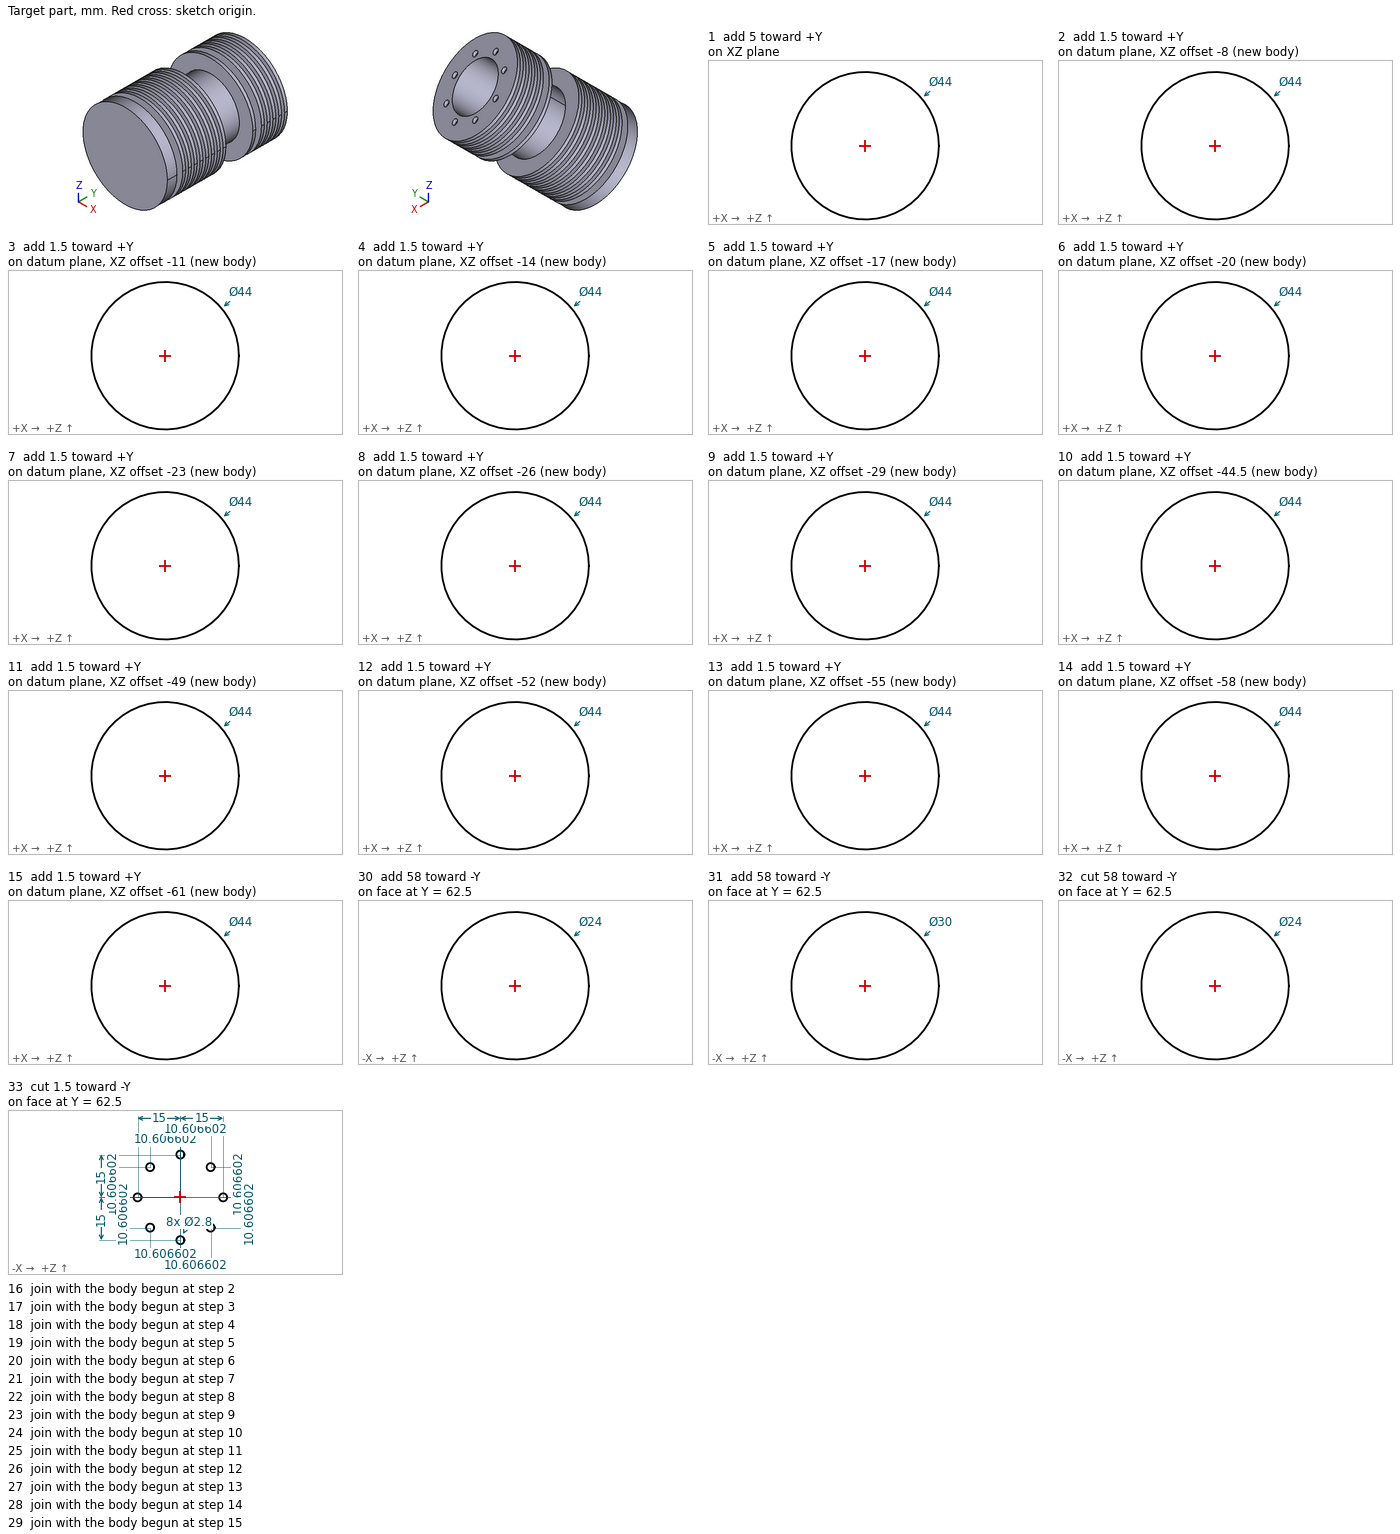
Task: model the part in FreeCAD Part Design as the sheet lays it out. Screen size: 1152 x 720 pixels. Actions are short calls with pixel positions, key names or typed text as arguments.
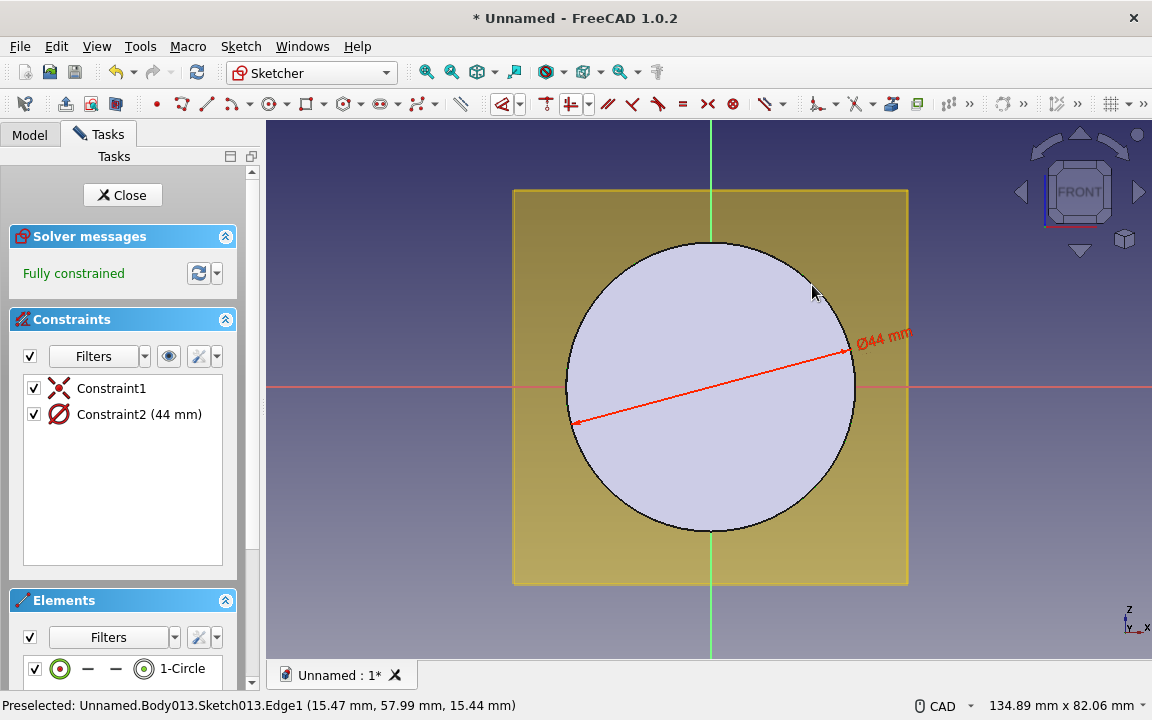
click(123, 195)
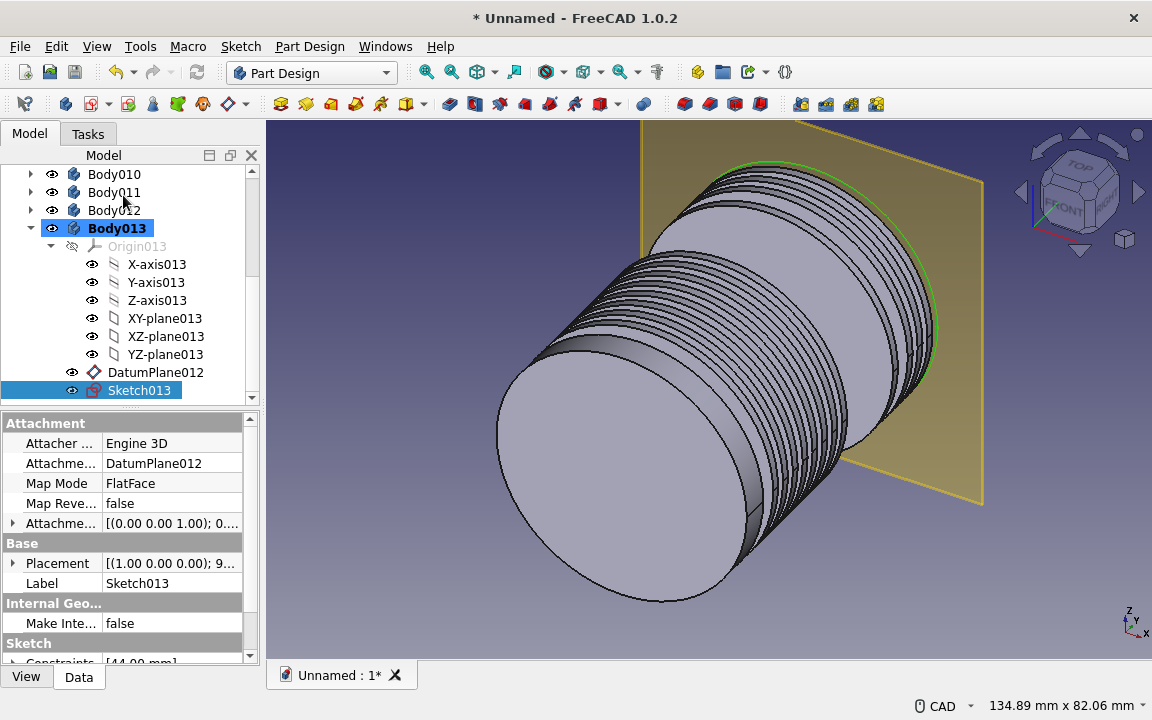
click(281, 104)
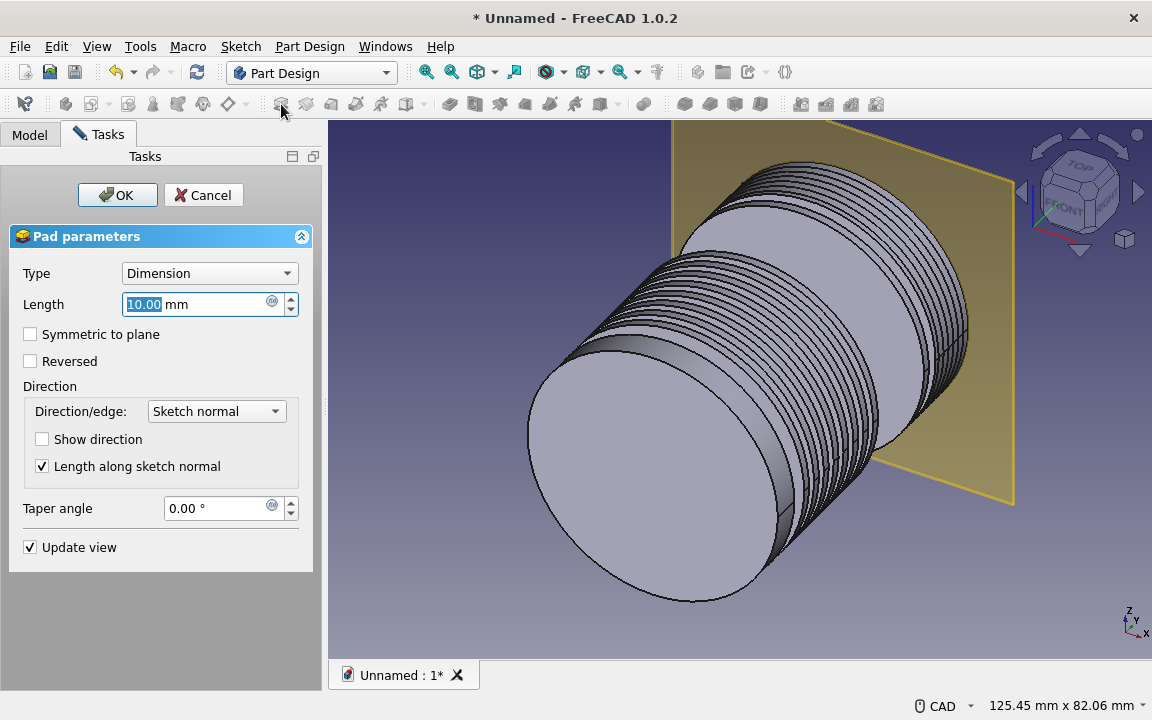
text(1.5)
key(Tab)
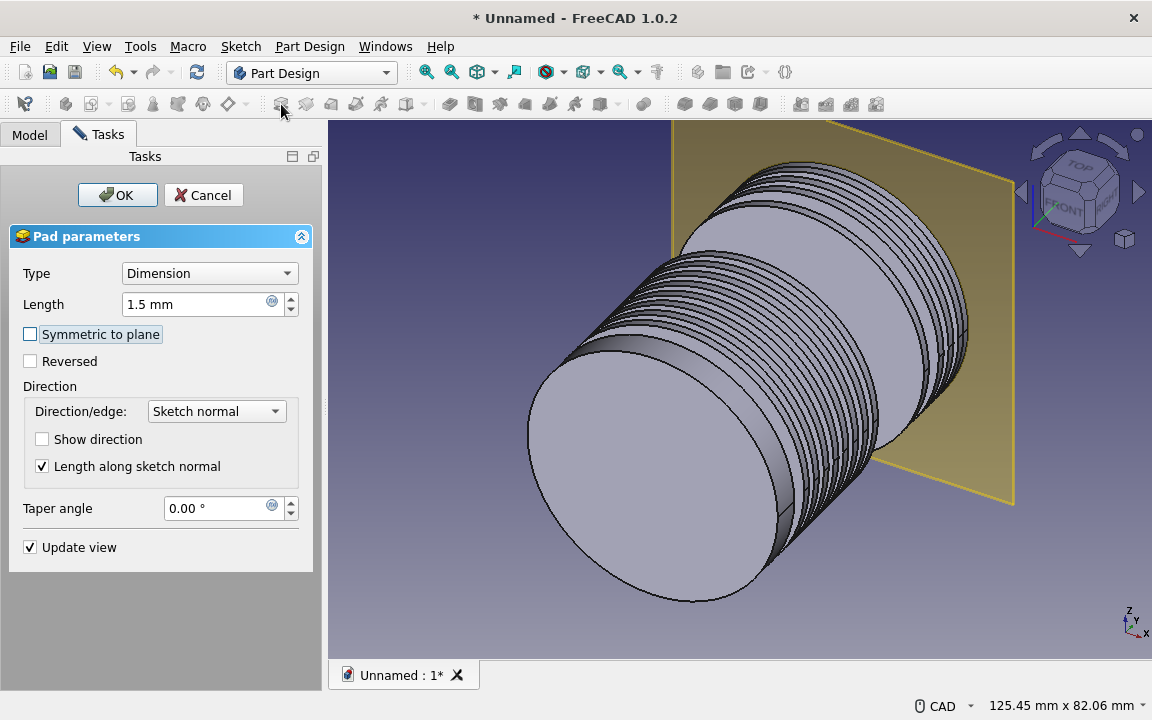
click(31, 361)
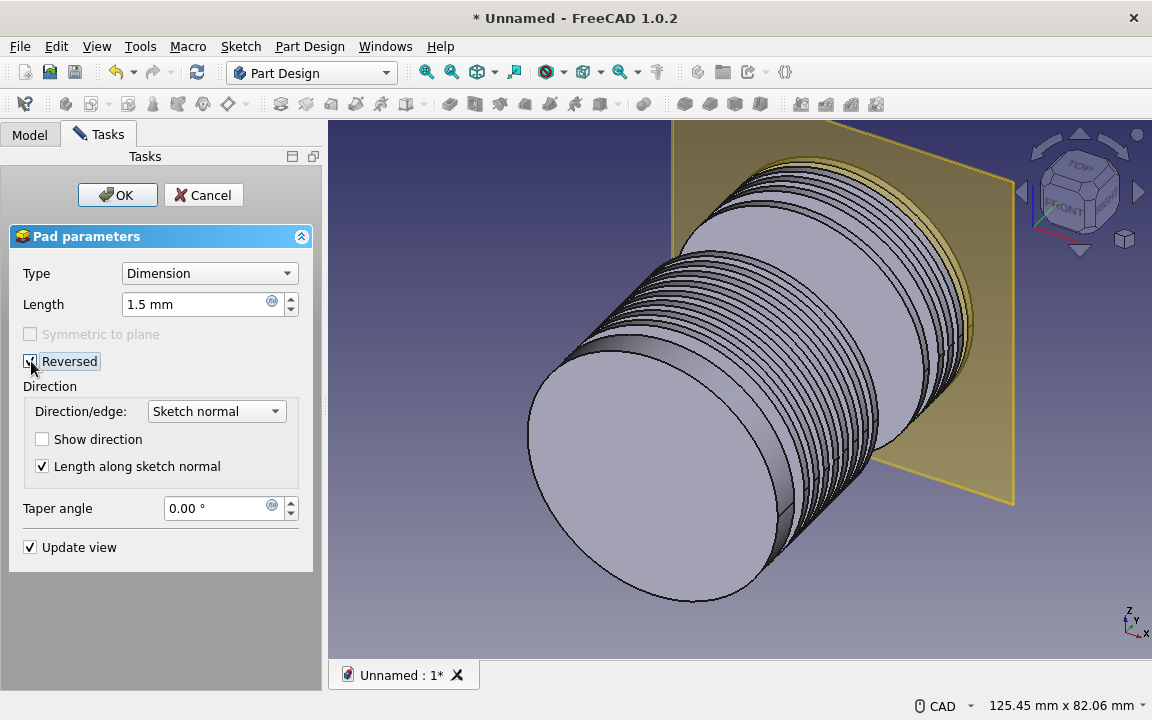
click(118, 195)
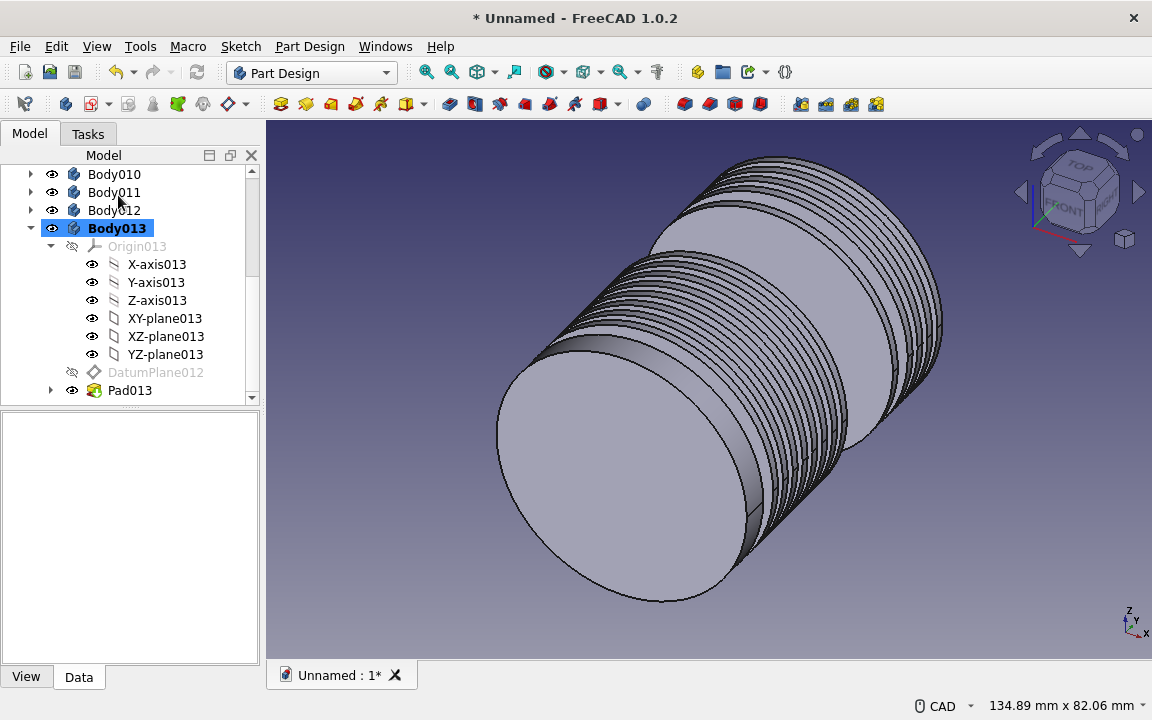
click(66, 104)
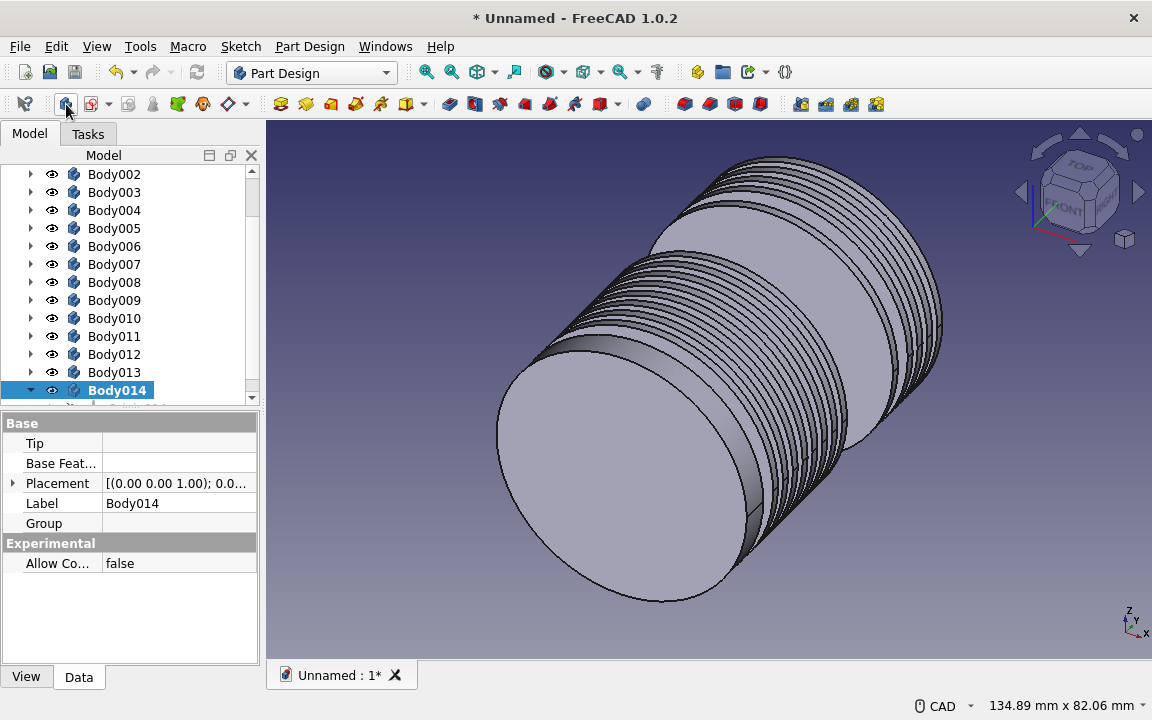
scroll(121, 278, down, 3)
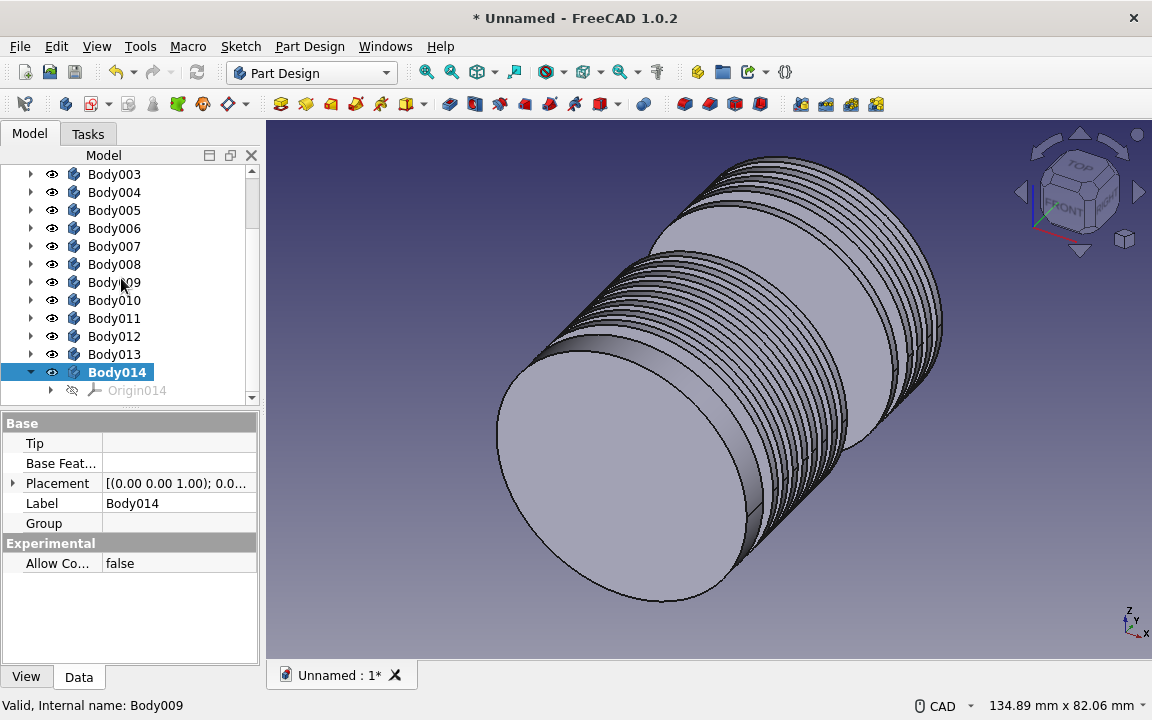
click(51, 390)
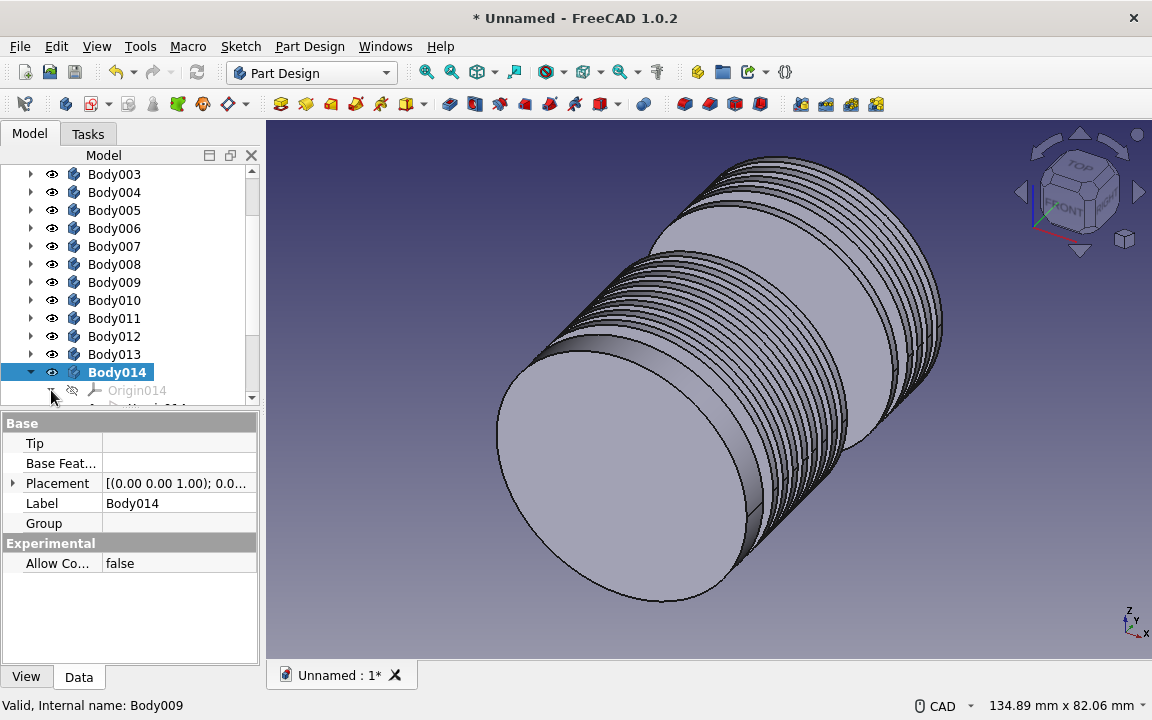
scroll(121, 278, down, 3)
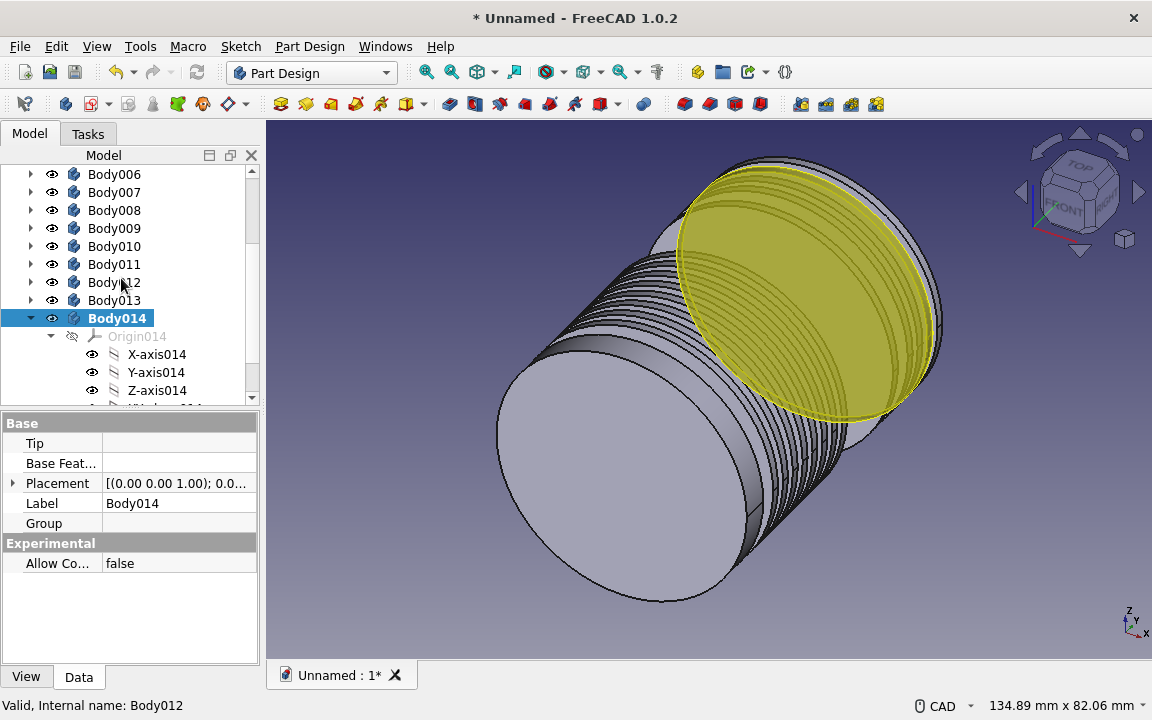
click(137, 372)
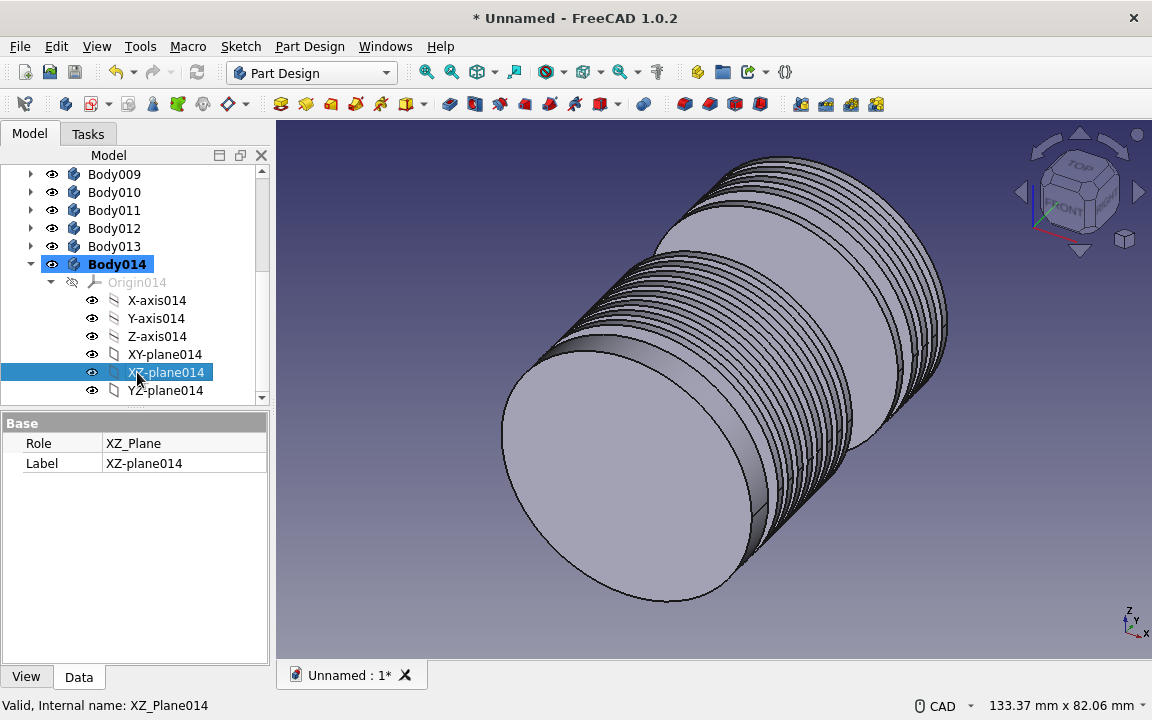
click(228, 104)